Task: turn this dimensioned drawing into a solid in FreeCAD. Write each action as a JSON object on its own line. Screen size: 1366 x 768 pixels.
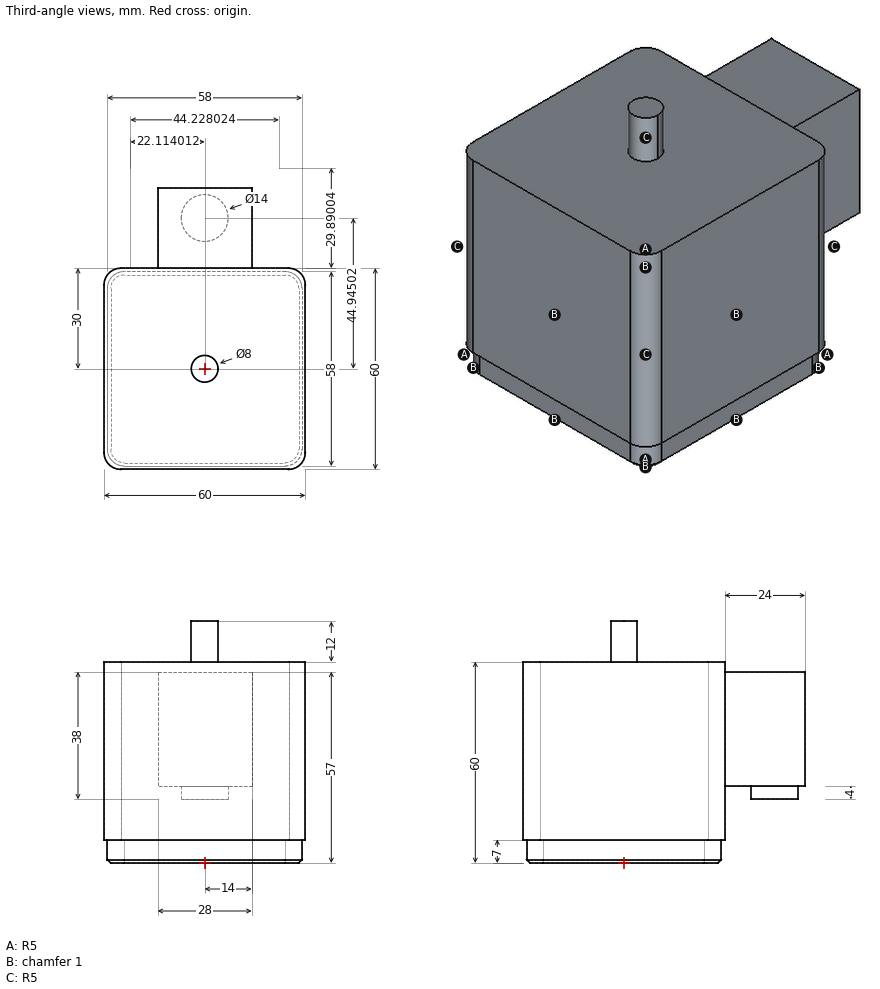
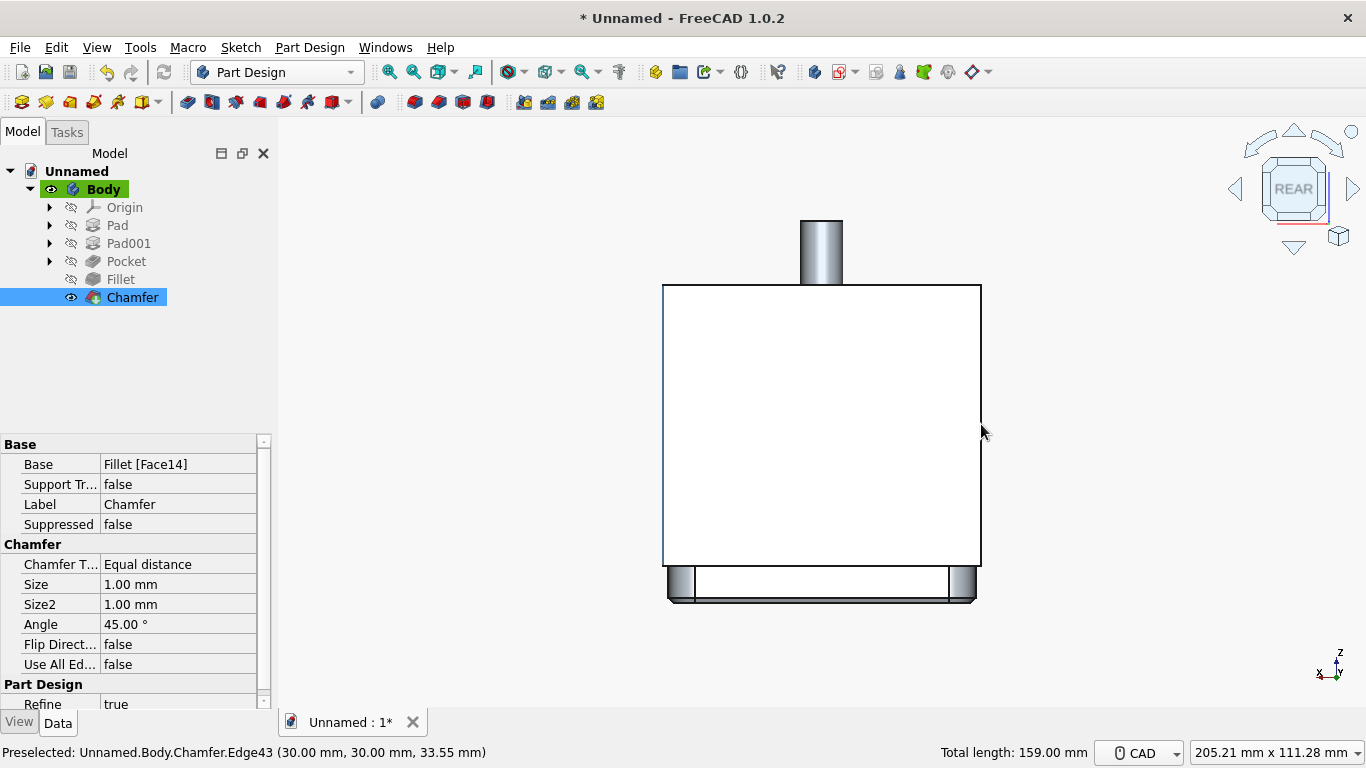
{"action": "left_click", "coordinate": [981, 424], "text": "ctrl"}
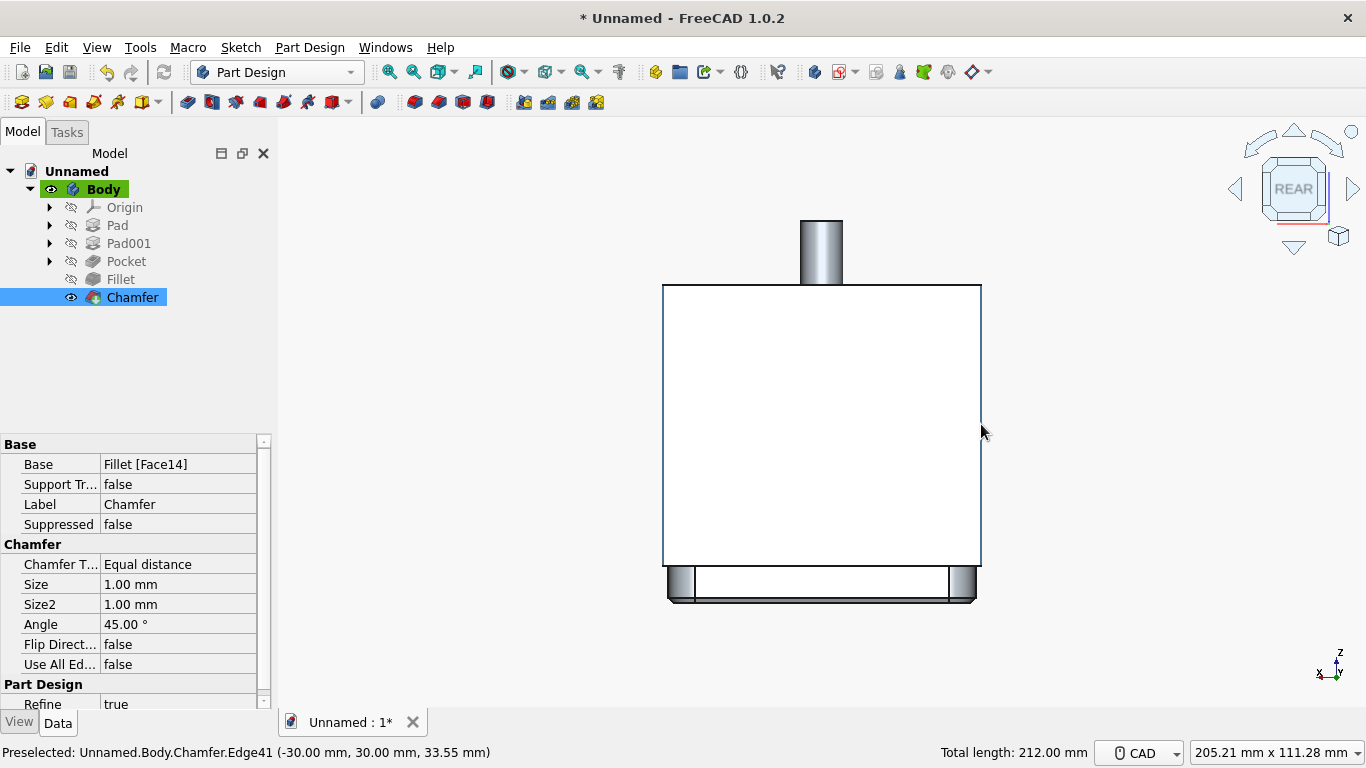
{"action": "left_click", "coordinate": [416, 102]}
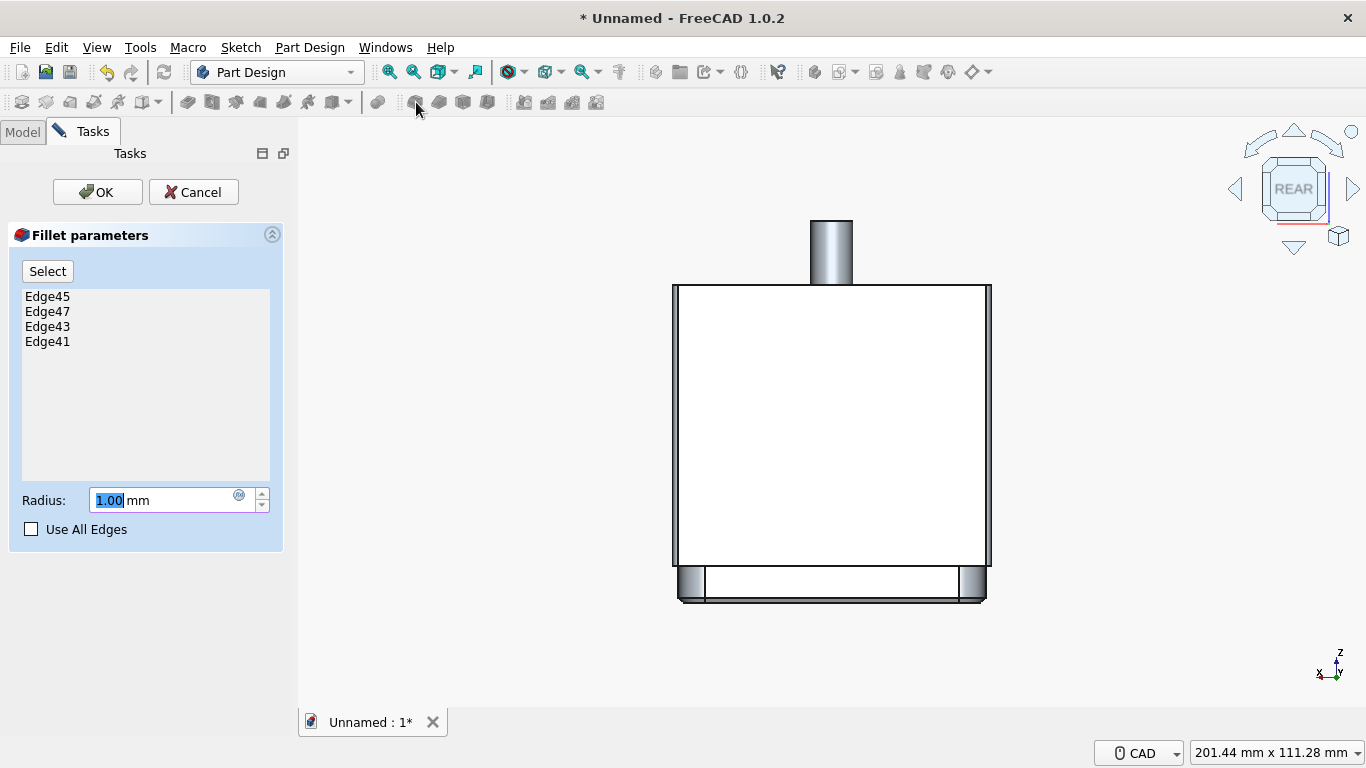
{"action": "type", "text": "5"}
{"action": "key", "text": "Tab"}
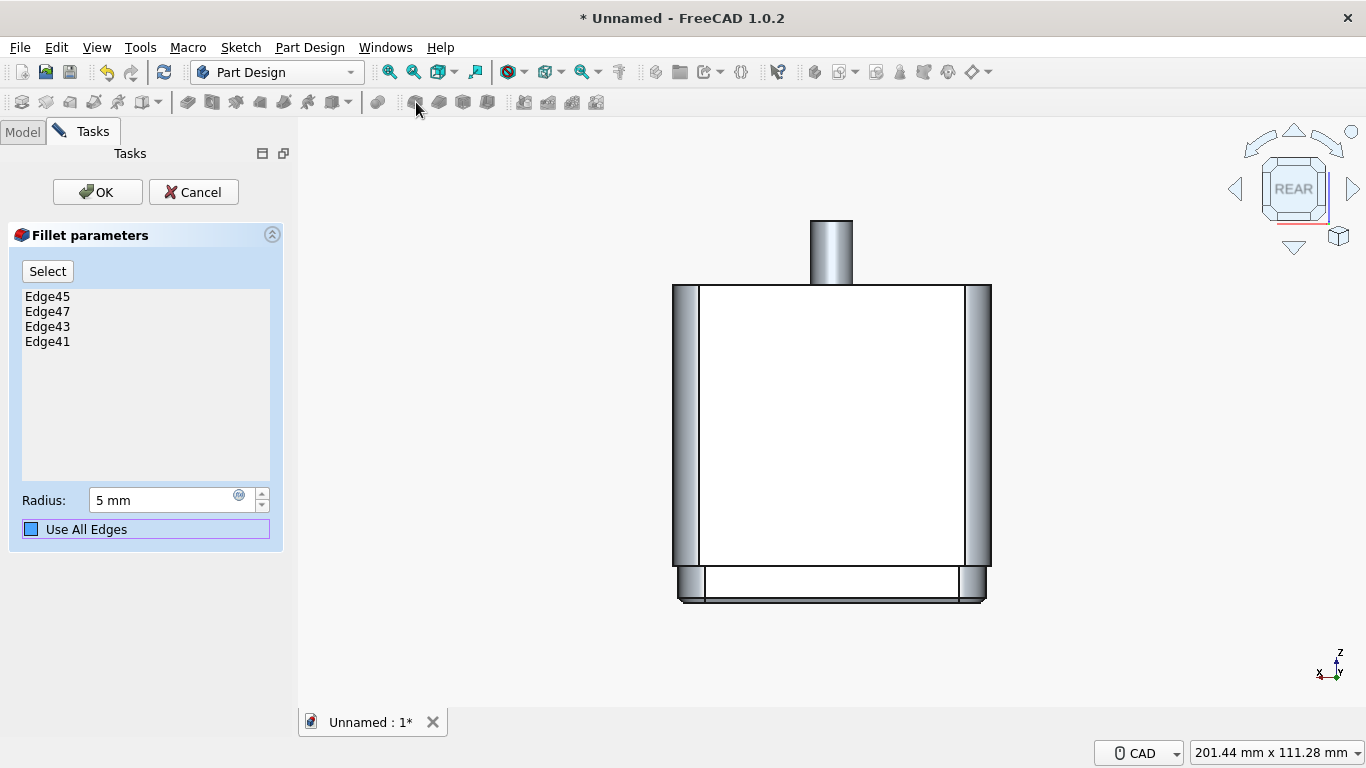
{"action": "left_click", "coordinate": [98, 192]}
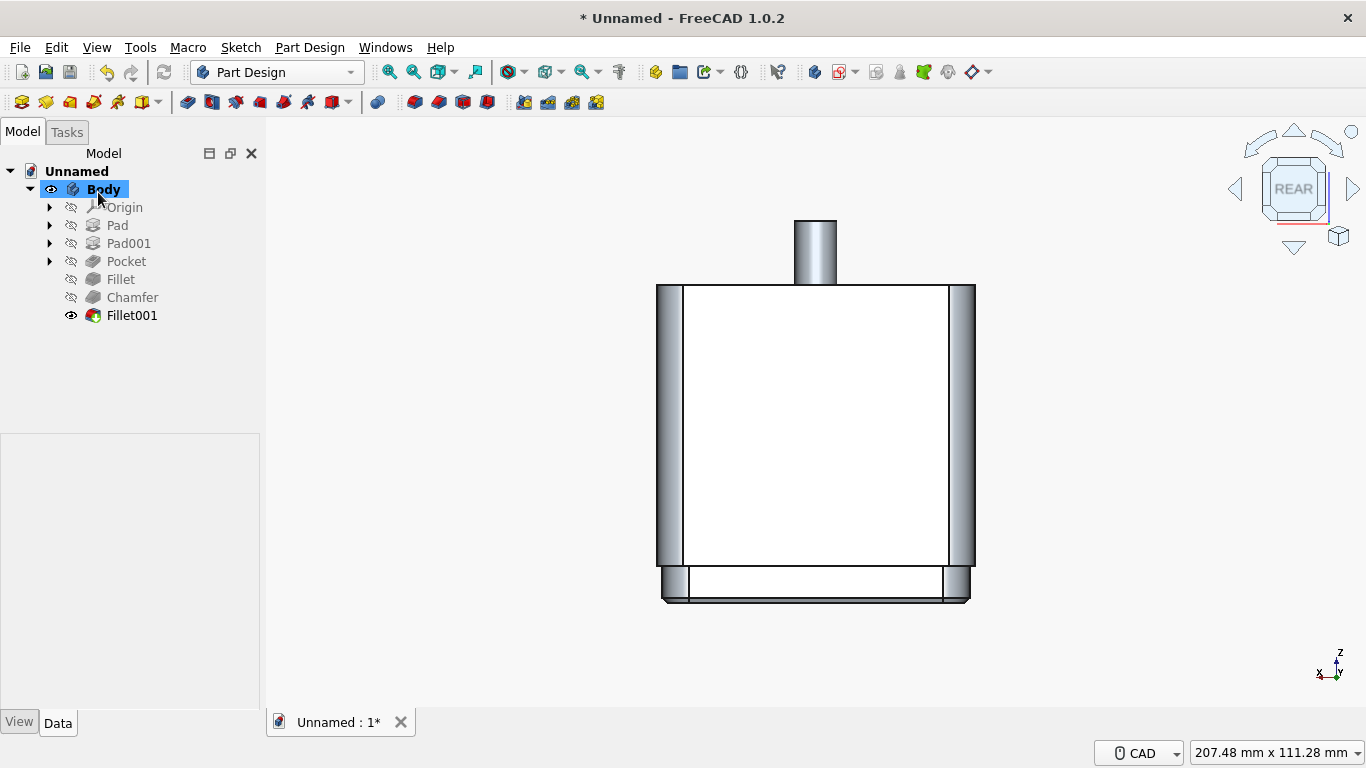
{"action": "left_click", "coordinate": [816, 424]}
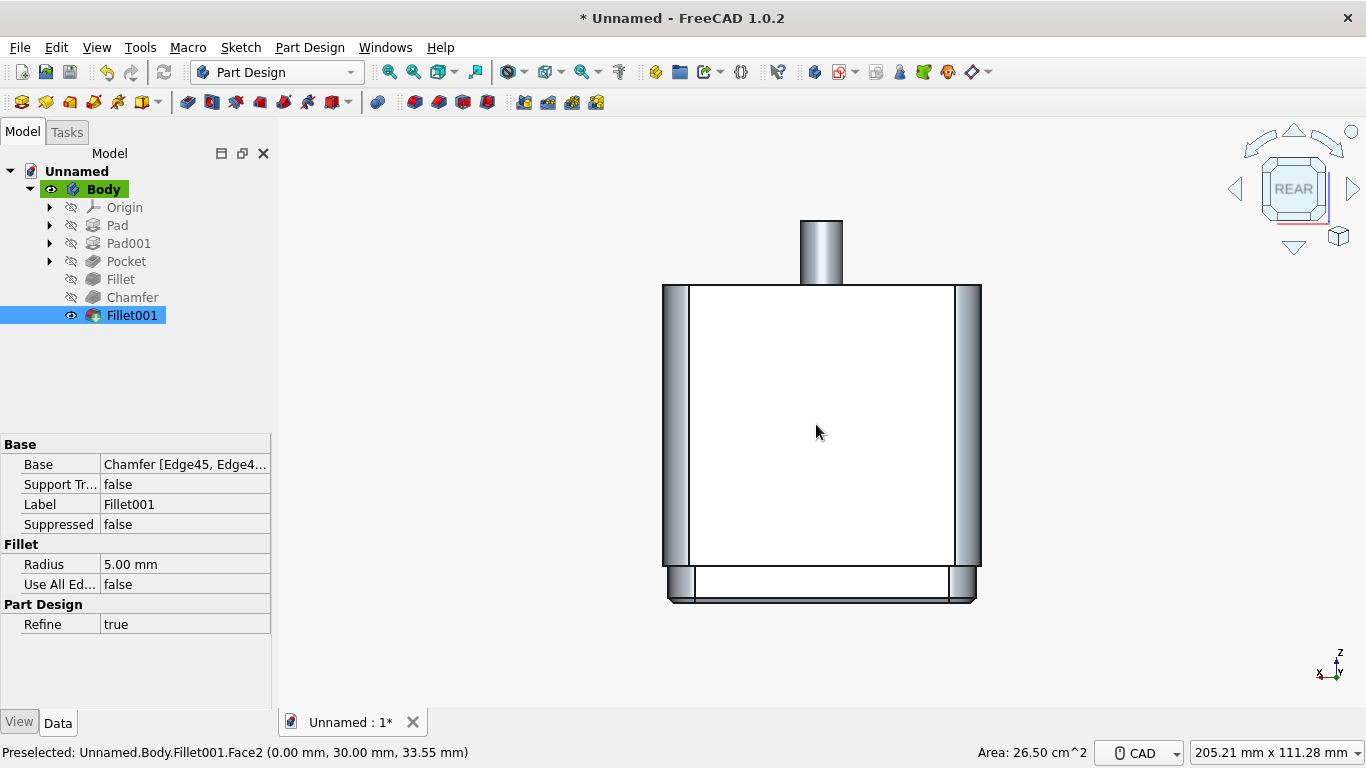
{"action": "left_click", "coordinate": [840, 72]}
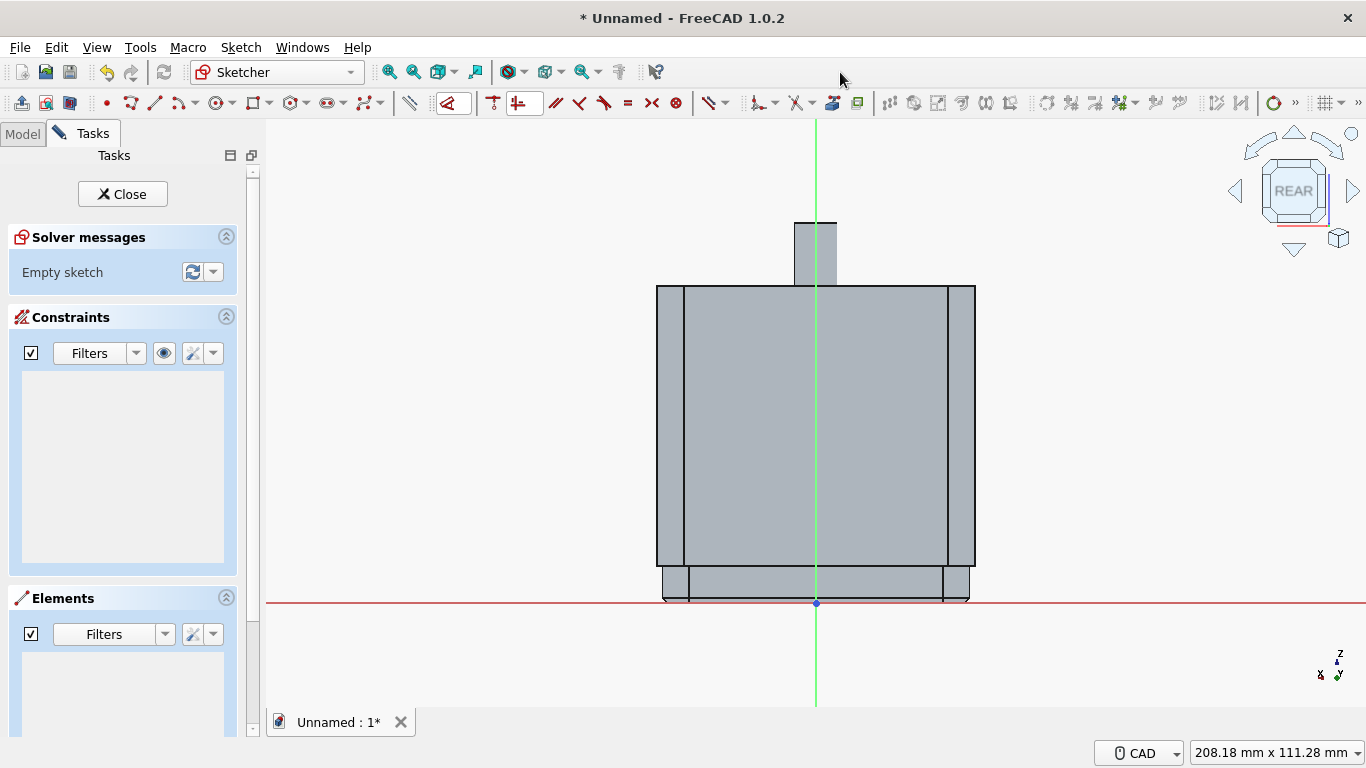
{"action": "key", "text": "g r"}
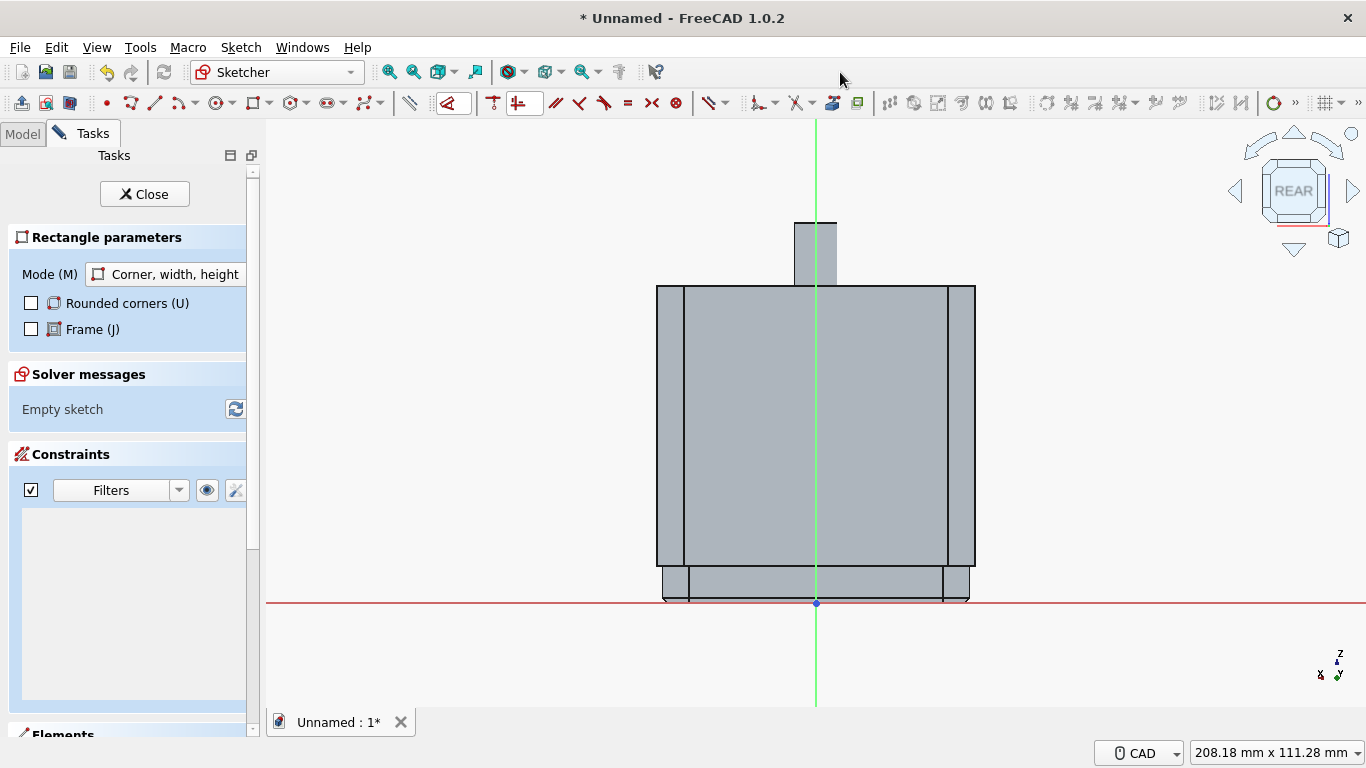
{"action": "left_click", "coordinate": [742, 302]}
{"action": "mouse_move", "coordinate": [890, 503]}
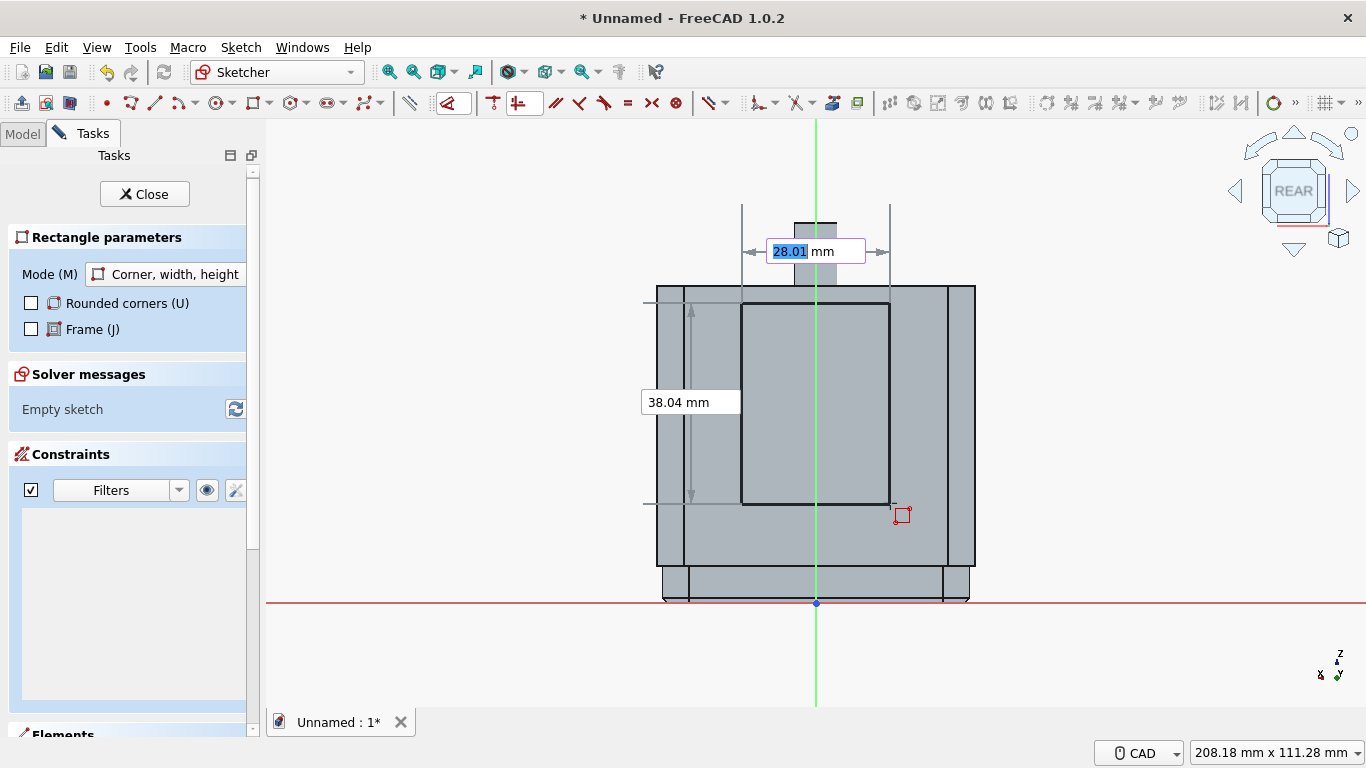
{"action": "type", "text": "28"}
{"action": "key", "text": "Tab"}
{"action": "type", "text": "38"}
{"action": "key", "text": "Return"}
{"action": "key", "text": "Escape"}